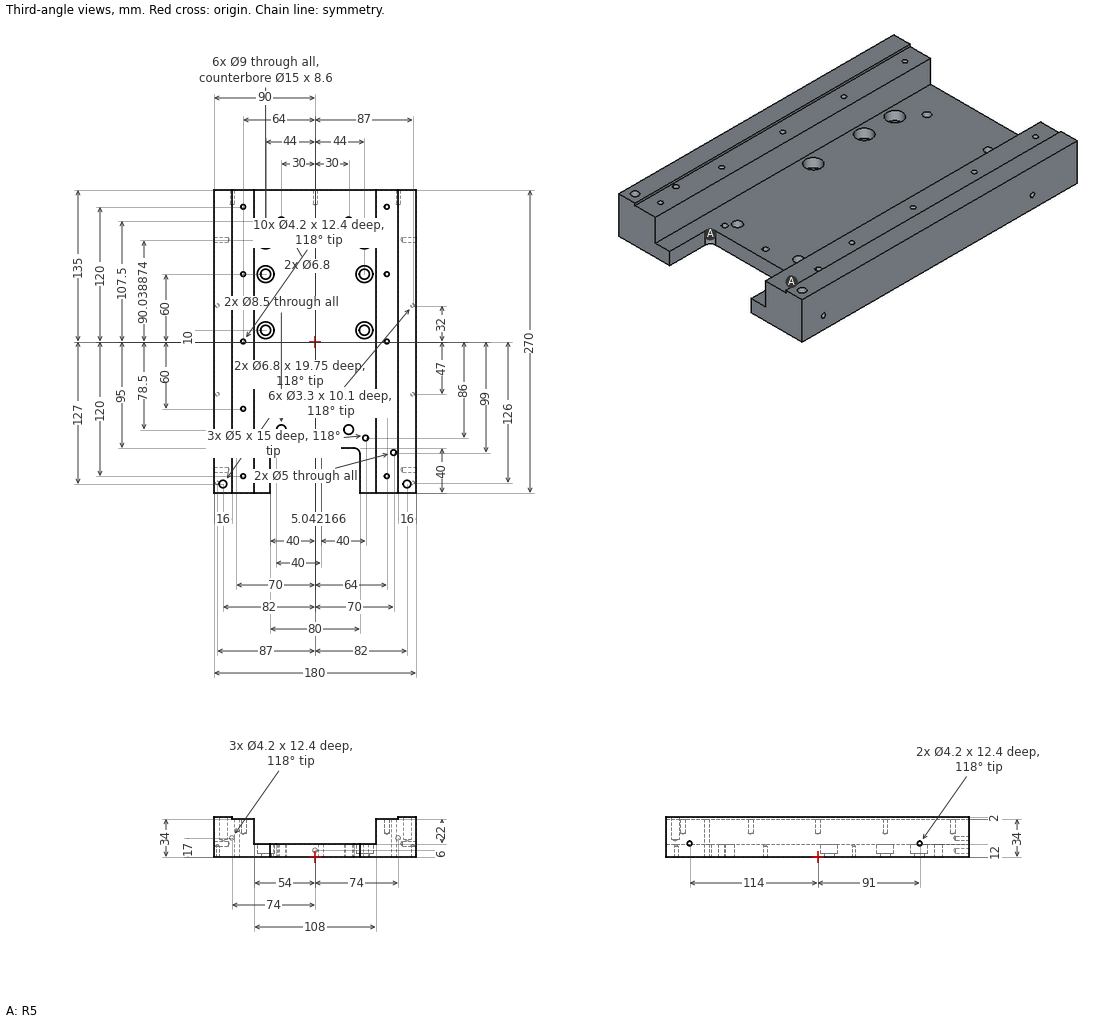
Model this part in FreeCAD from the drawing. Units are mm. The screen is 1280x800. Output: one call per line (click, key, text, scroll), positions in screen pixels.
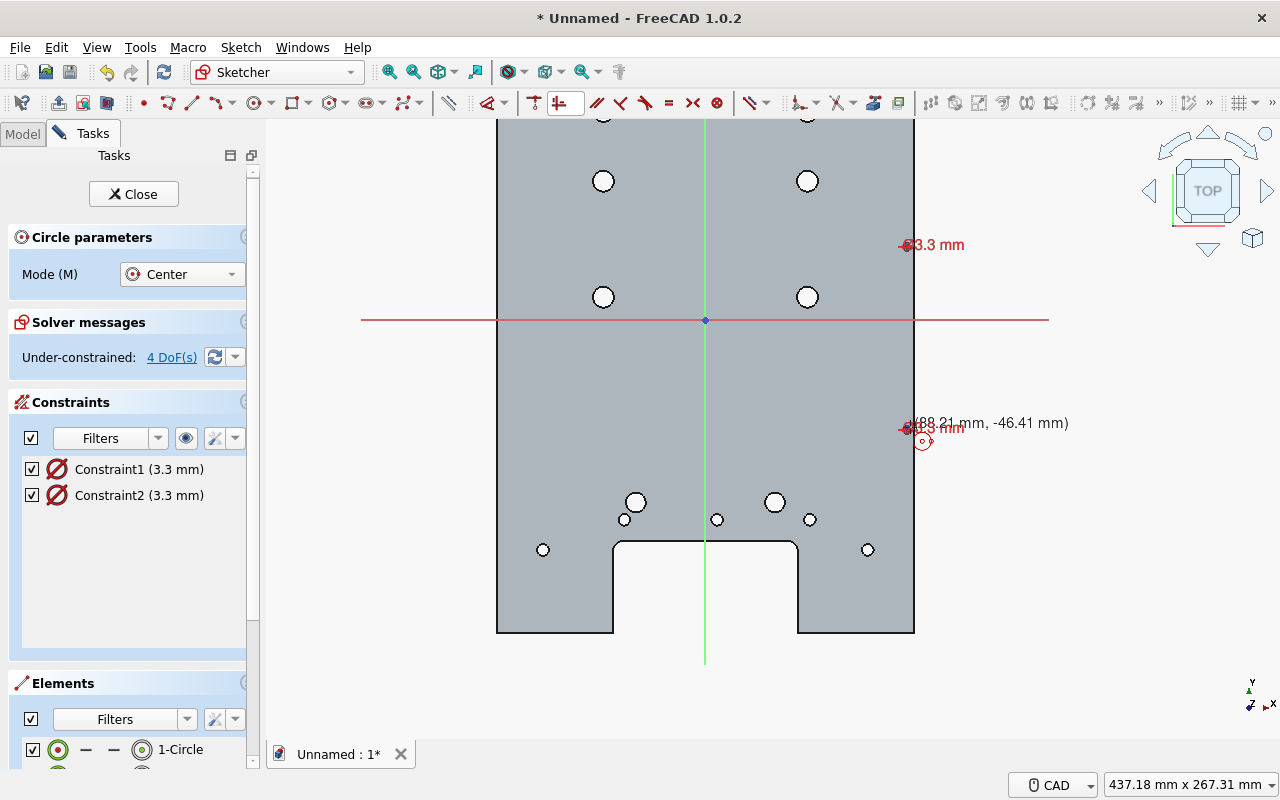
scroll(907, 613, up, 9)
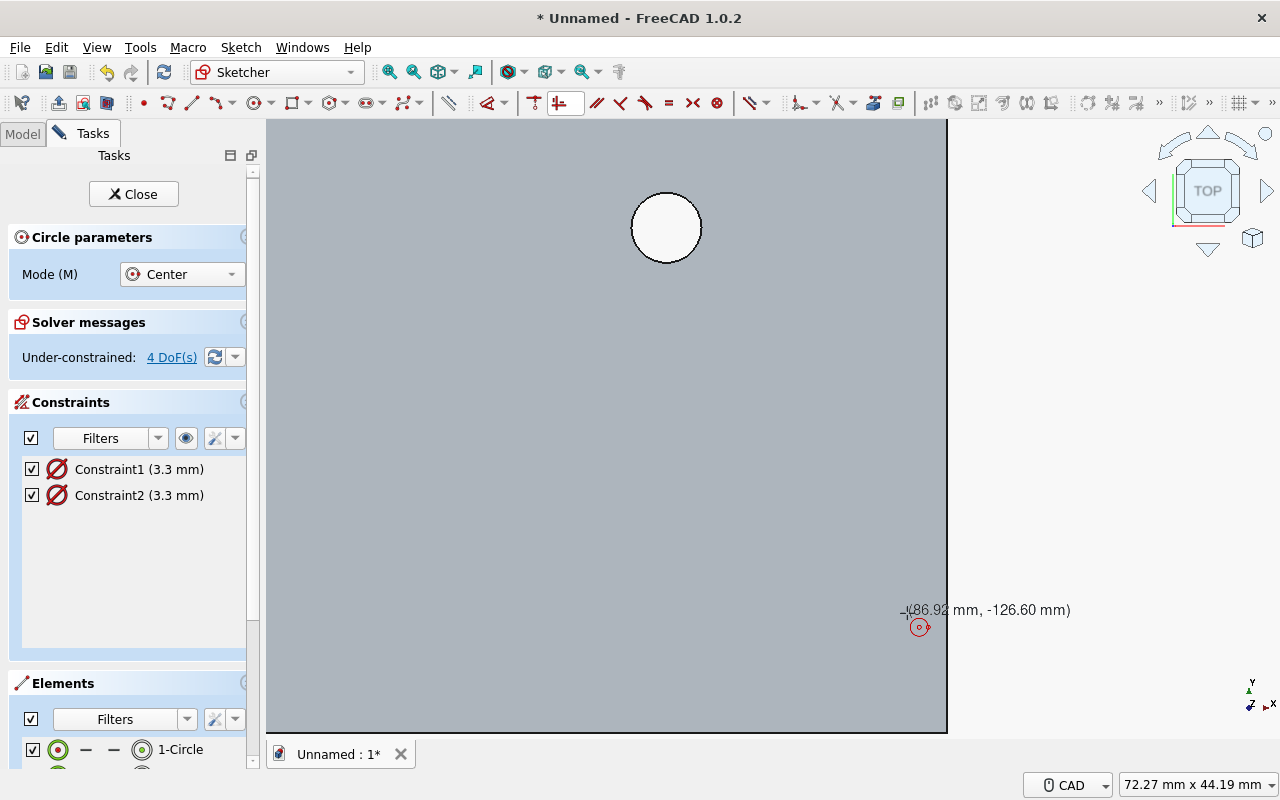
scroll(907, 613, down, 9)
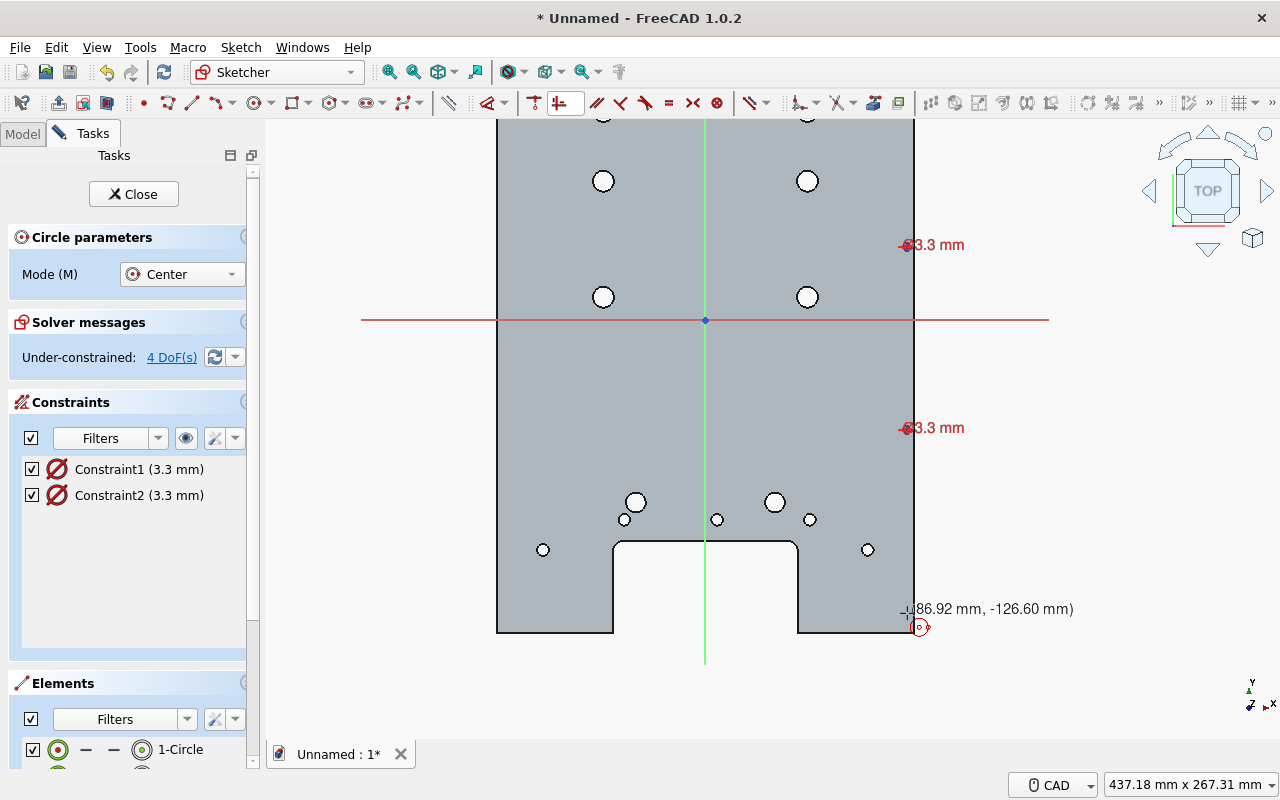
click(907, 613)
move(910, 610)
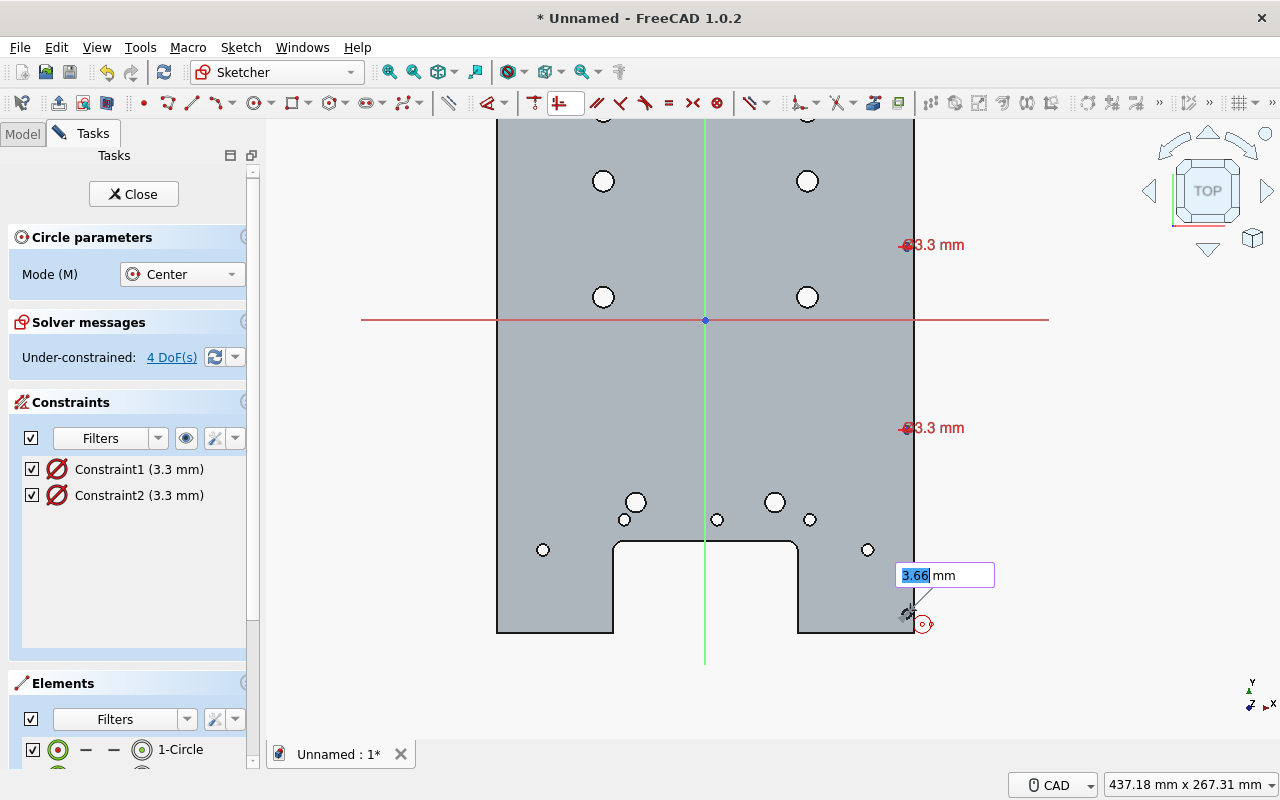
text(3.3)
key(Return)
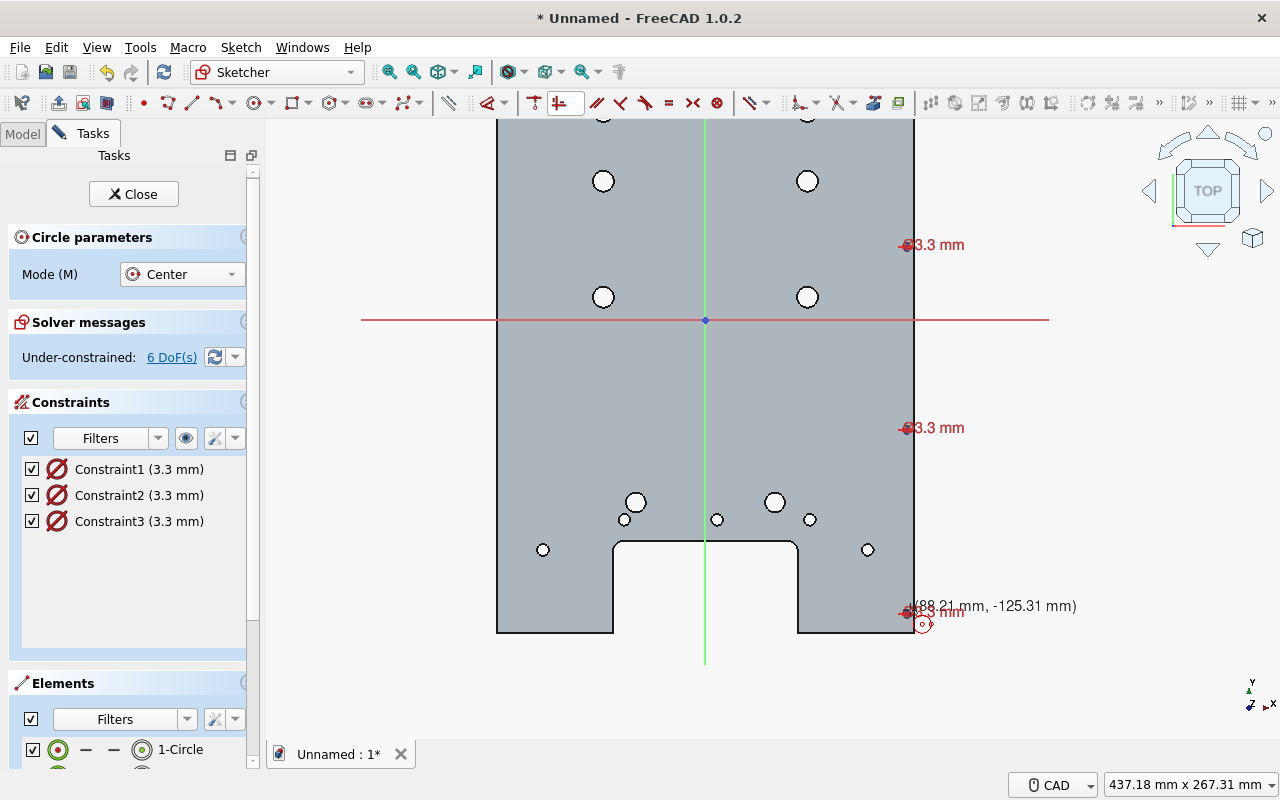
scroll(504, 613, up, 9)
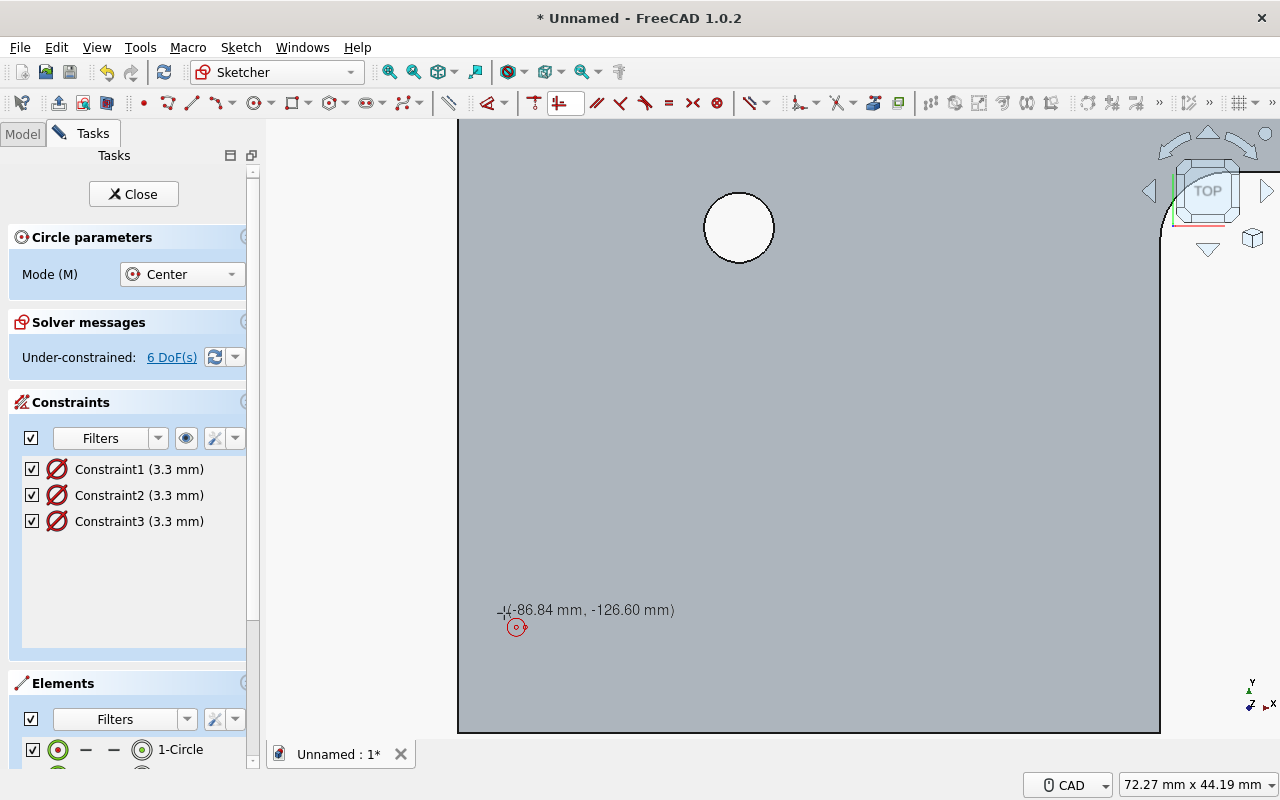
scroll(503, 613, down, 9)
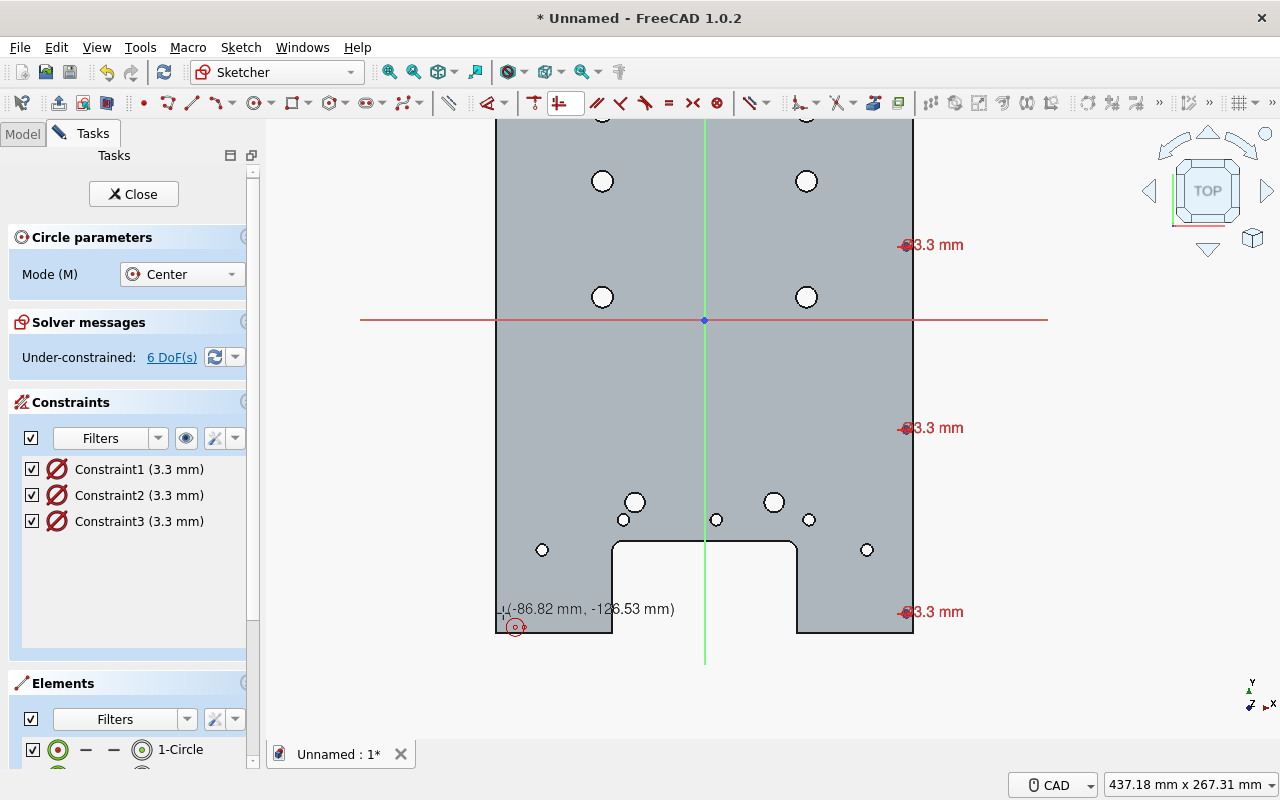
click(503, 613)
move(505, 610)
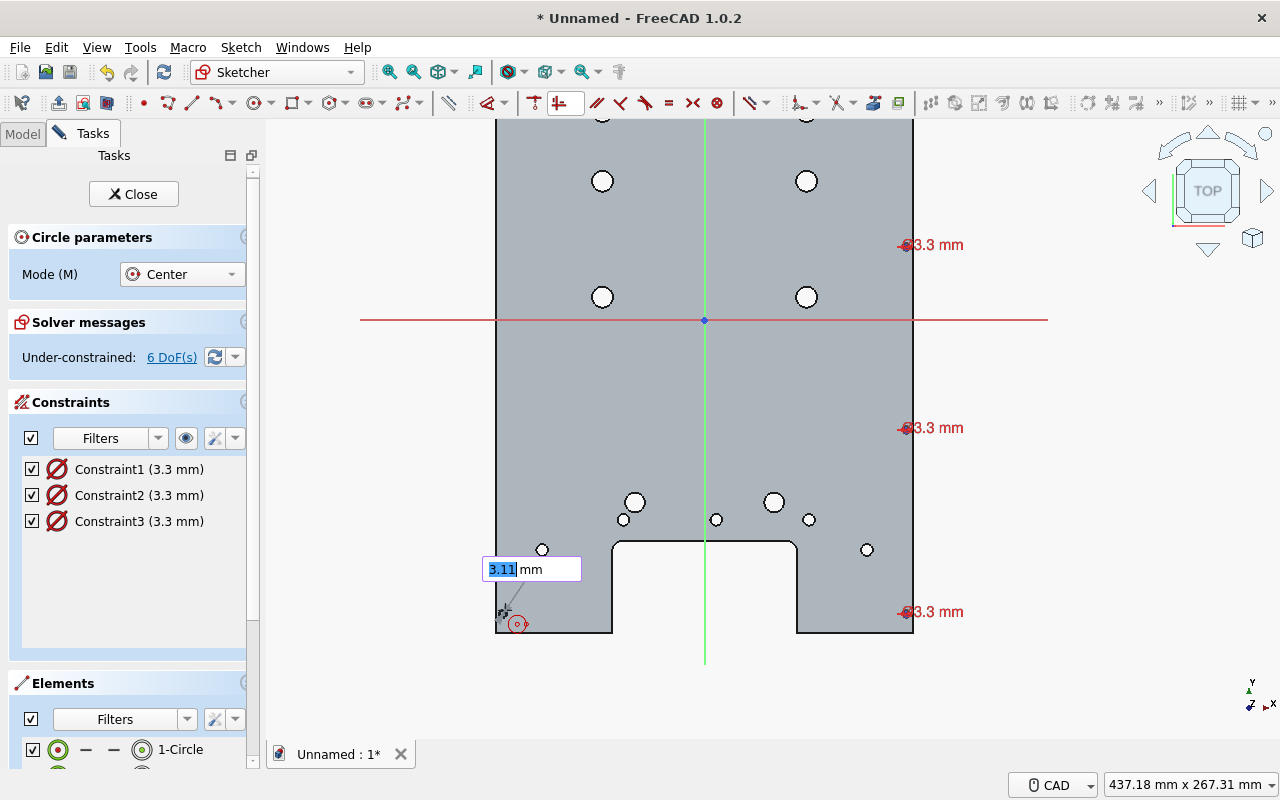
text(3.3)
key(Return)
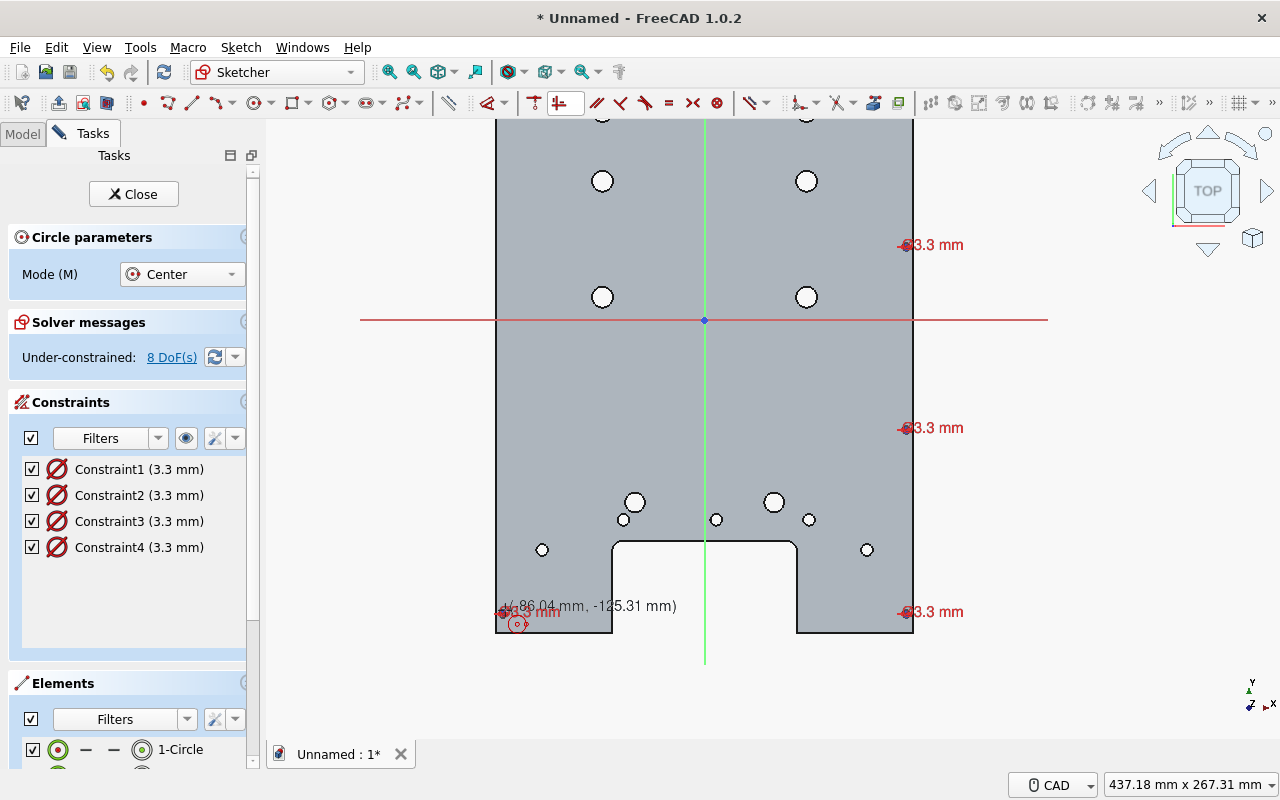
scroll(503, 429, up, 9)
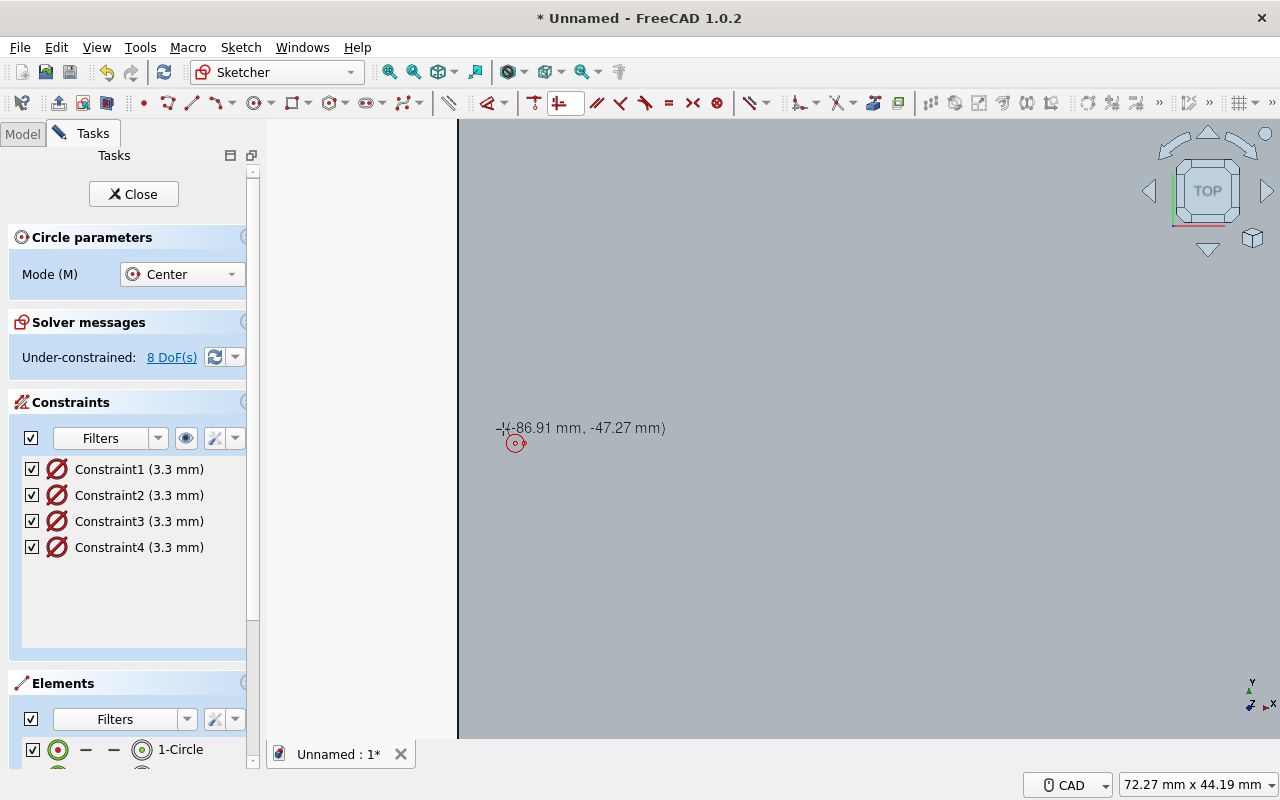
scroll(503, 429, down, 9)